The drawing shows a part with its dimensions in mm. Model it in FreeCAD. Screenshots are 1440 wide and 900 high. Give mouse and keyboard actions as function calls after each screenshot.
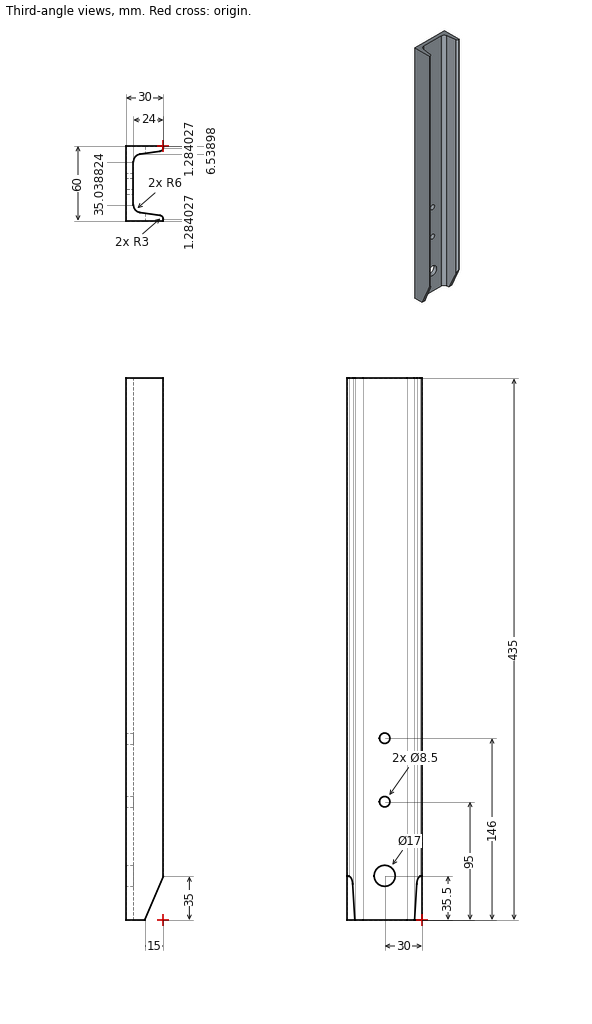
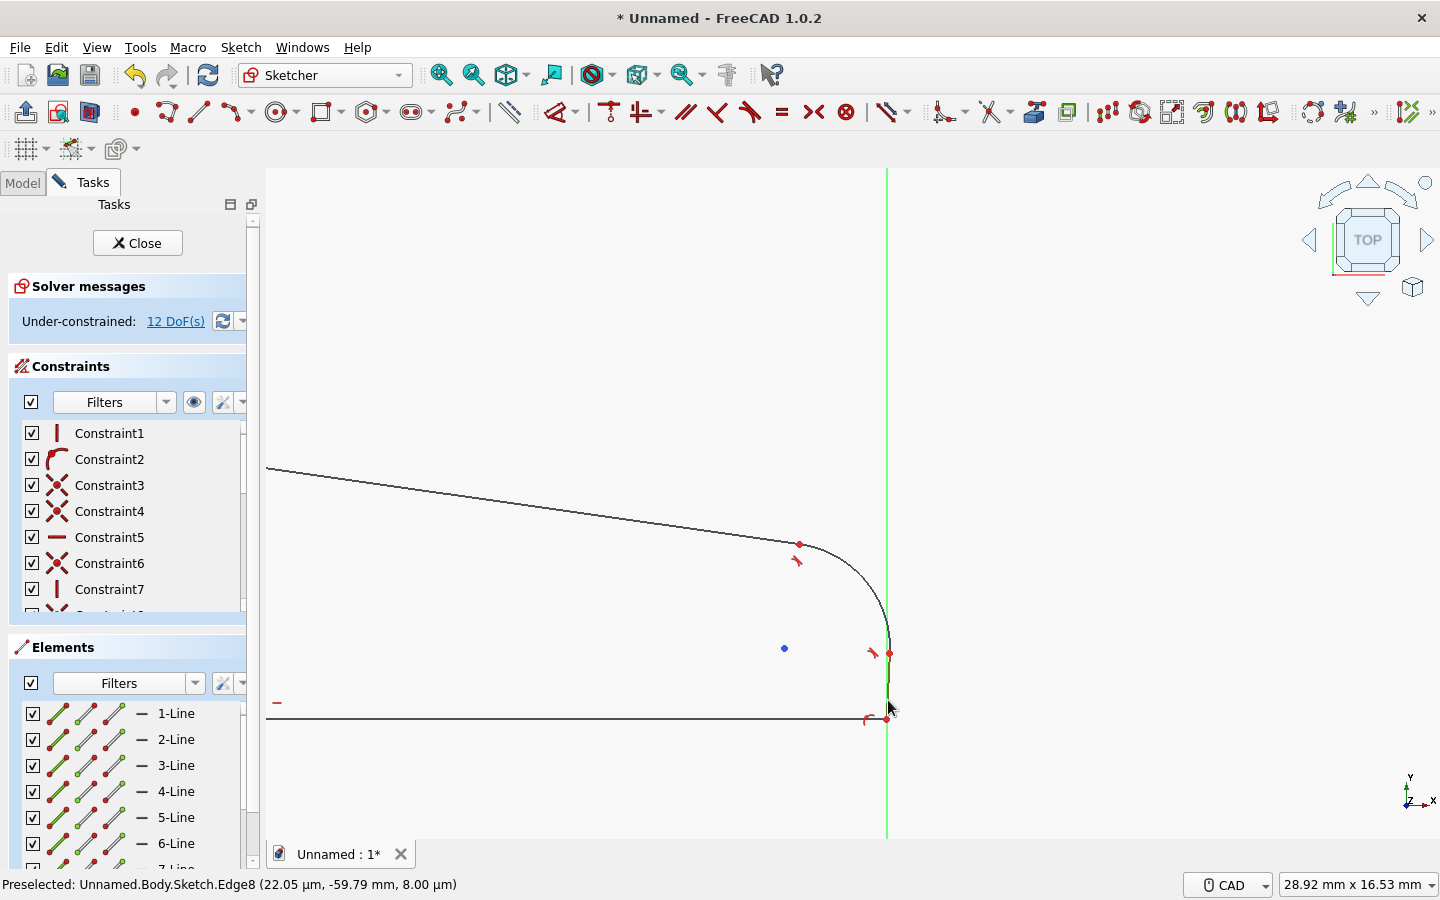
key(v)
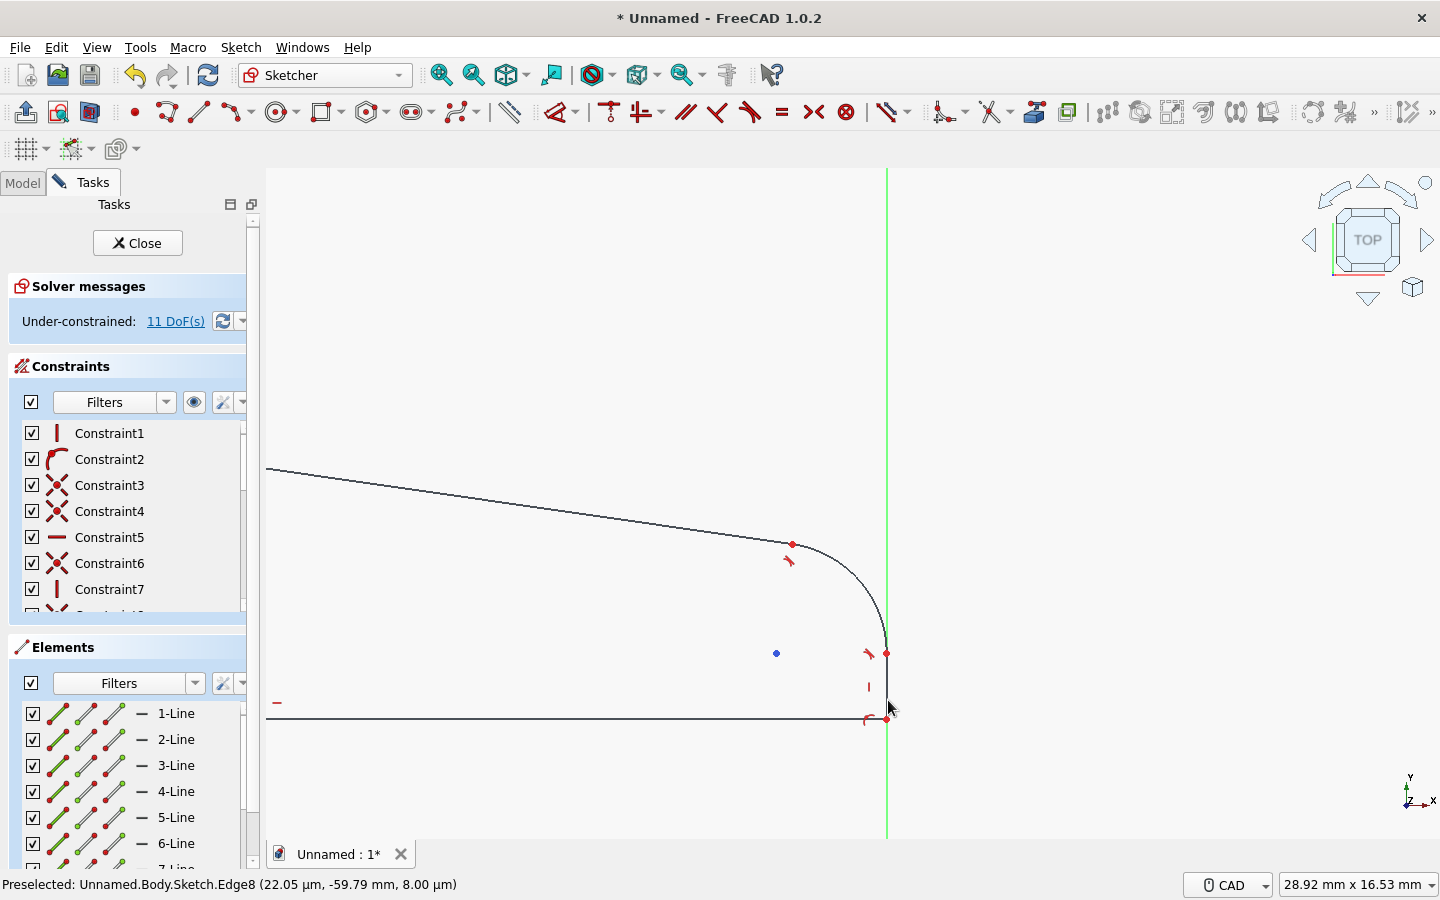
scroll(885, 704, down, 9)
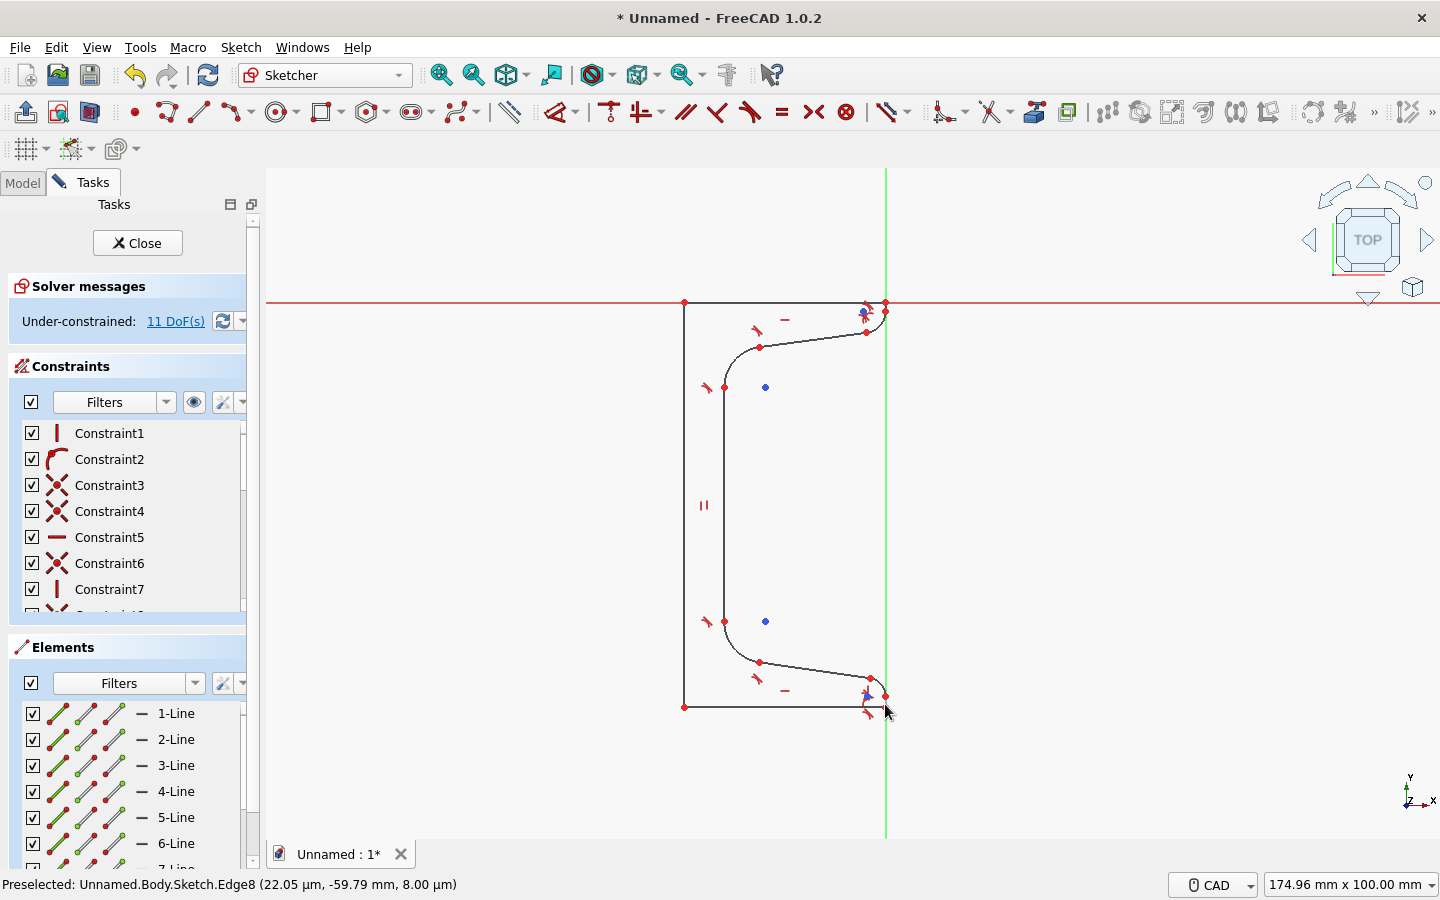
click(728, 639)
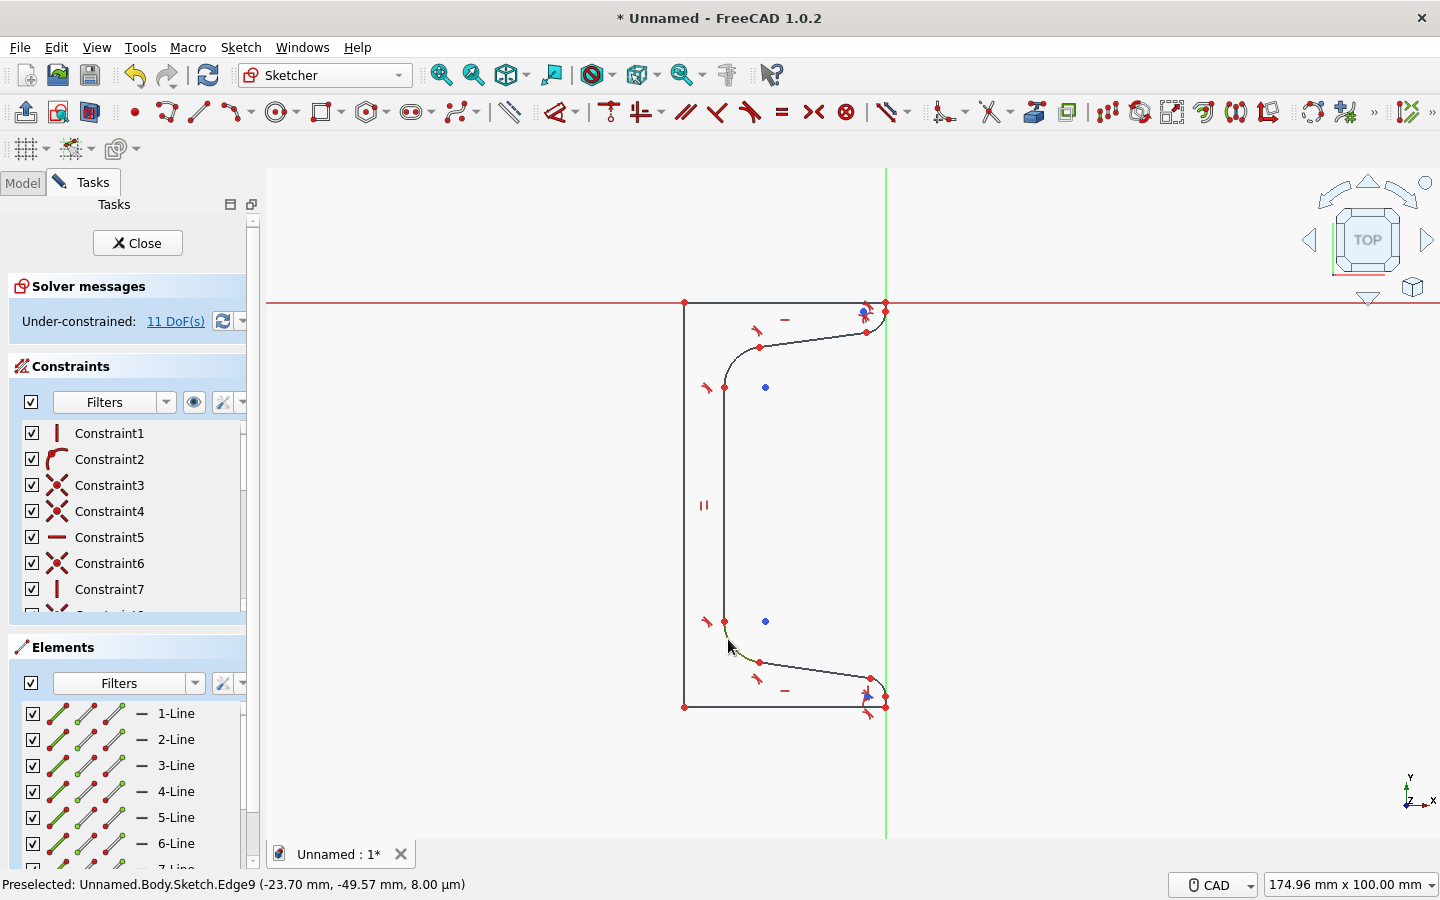
click(743, 353)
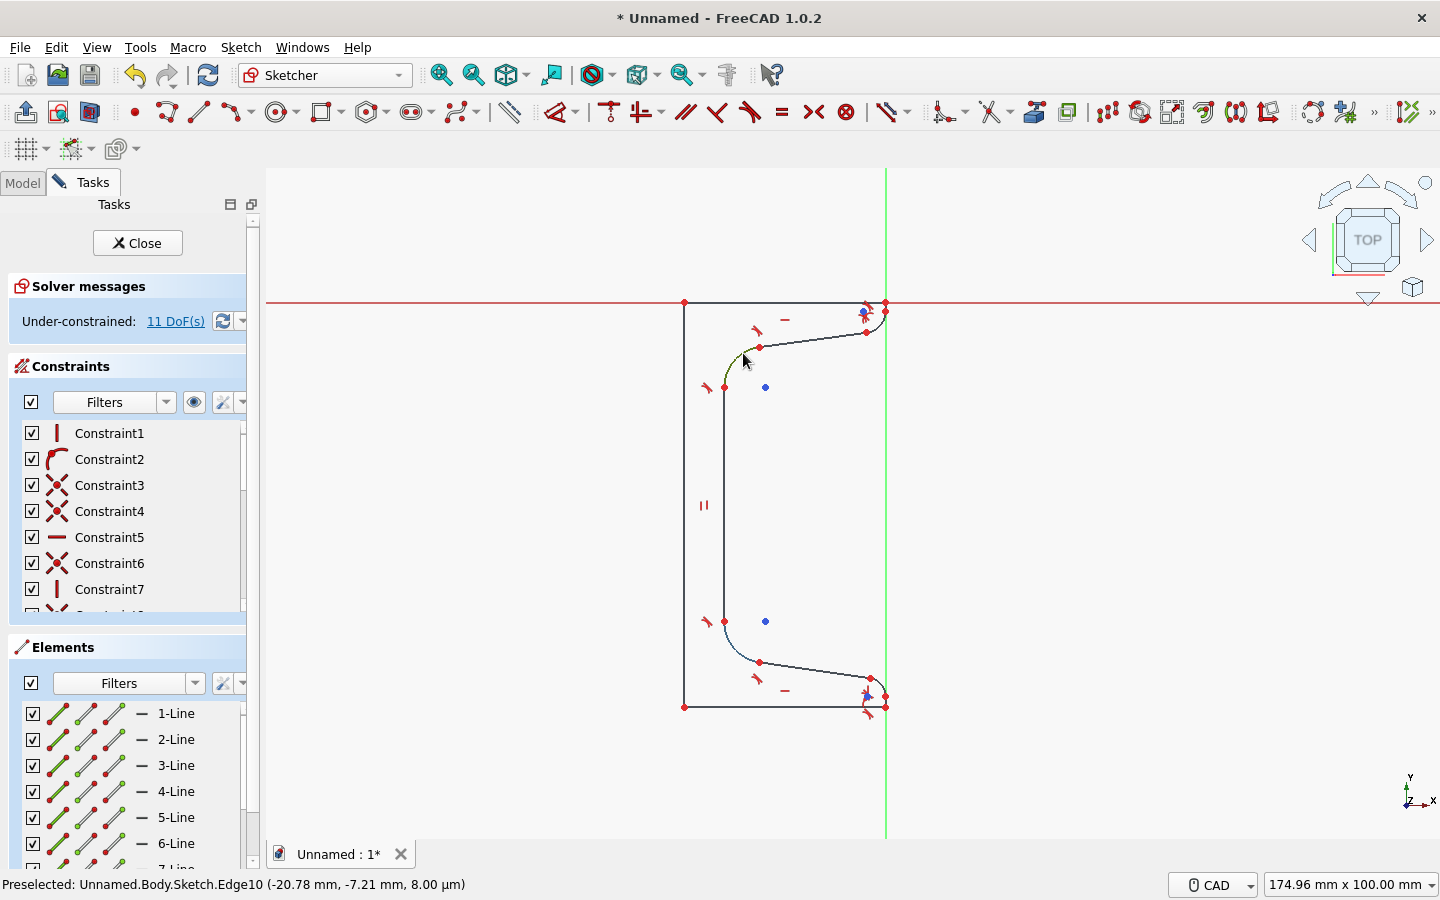
key(e)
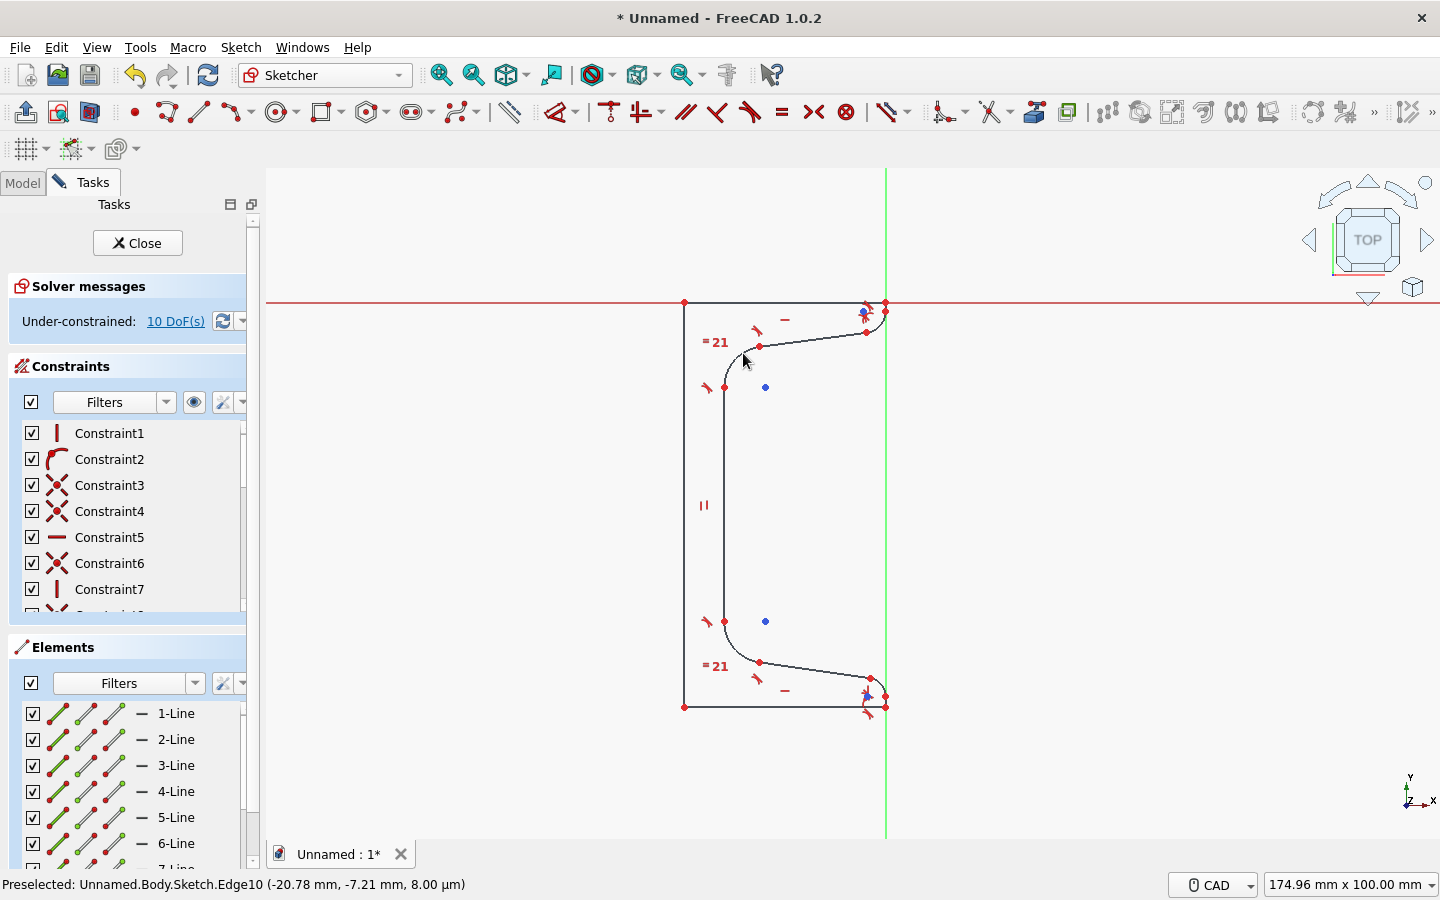
scroll(875, 330, up, 2)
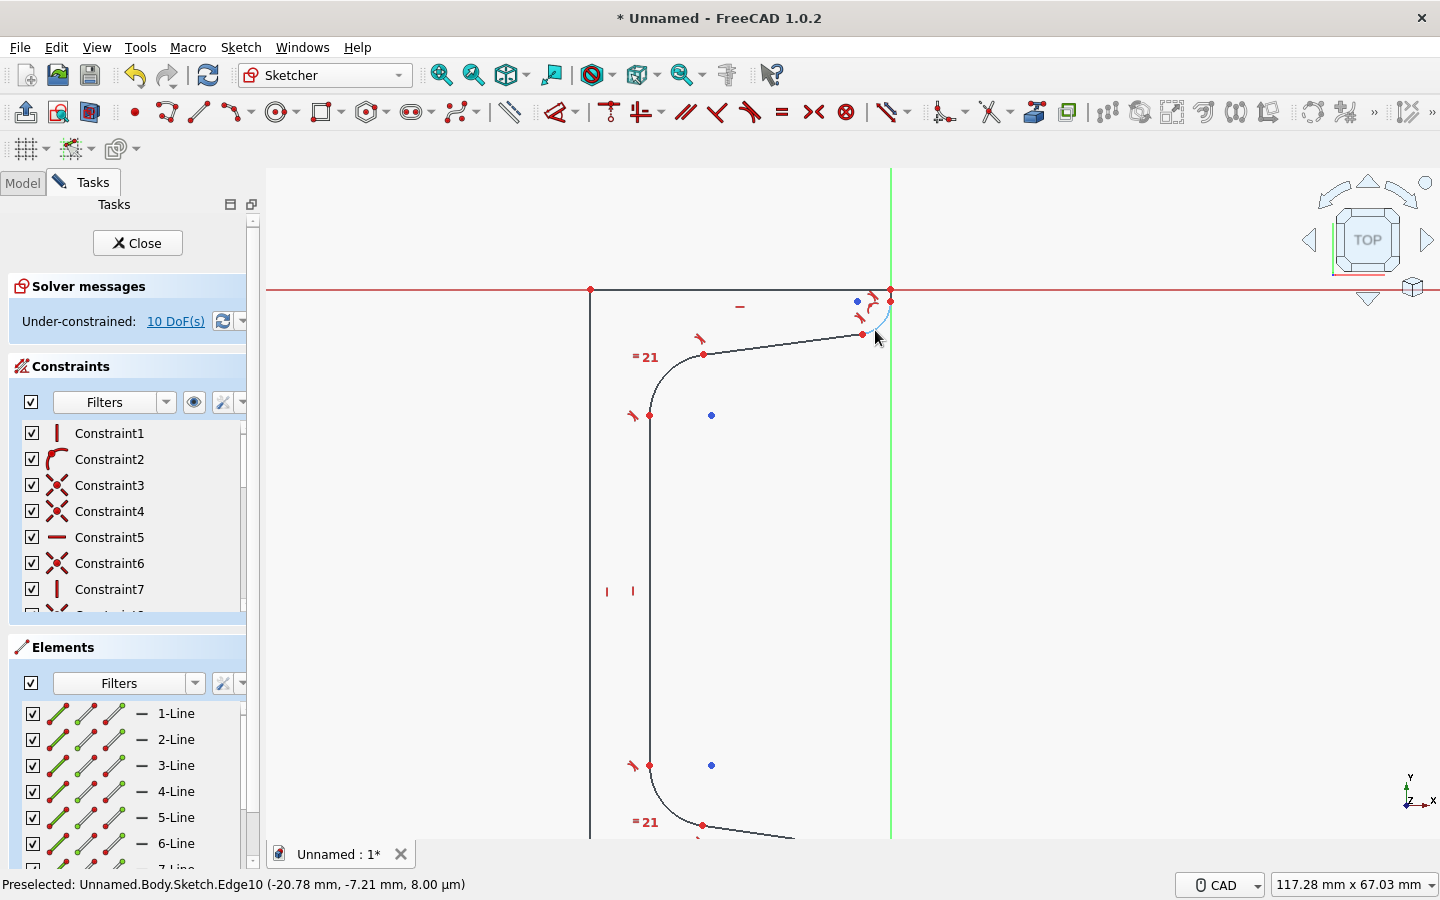
click(875, 329)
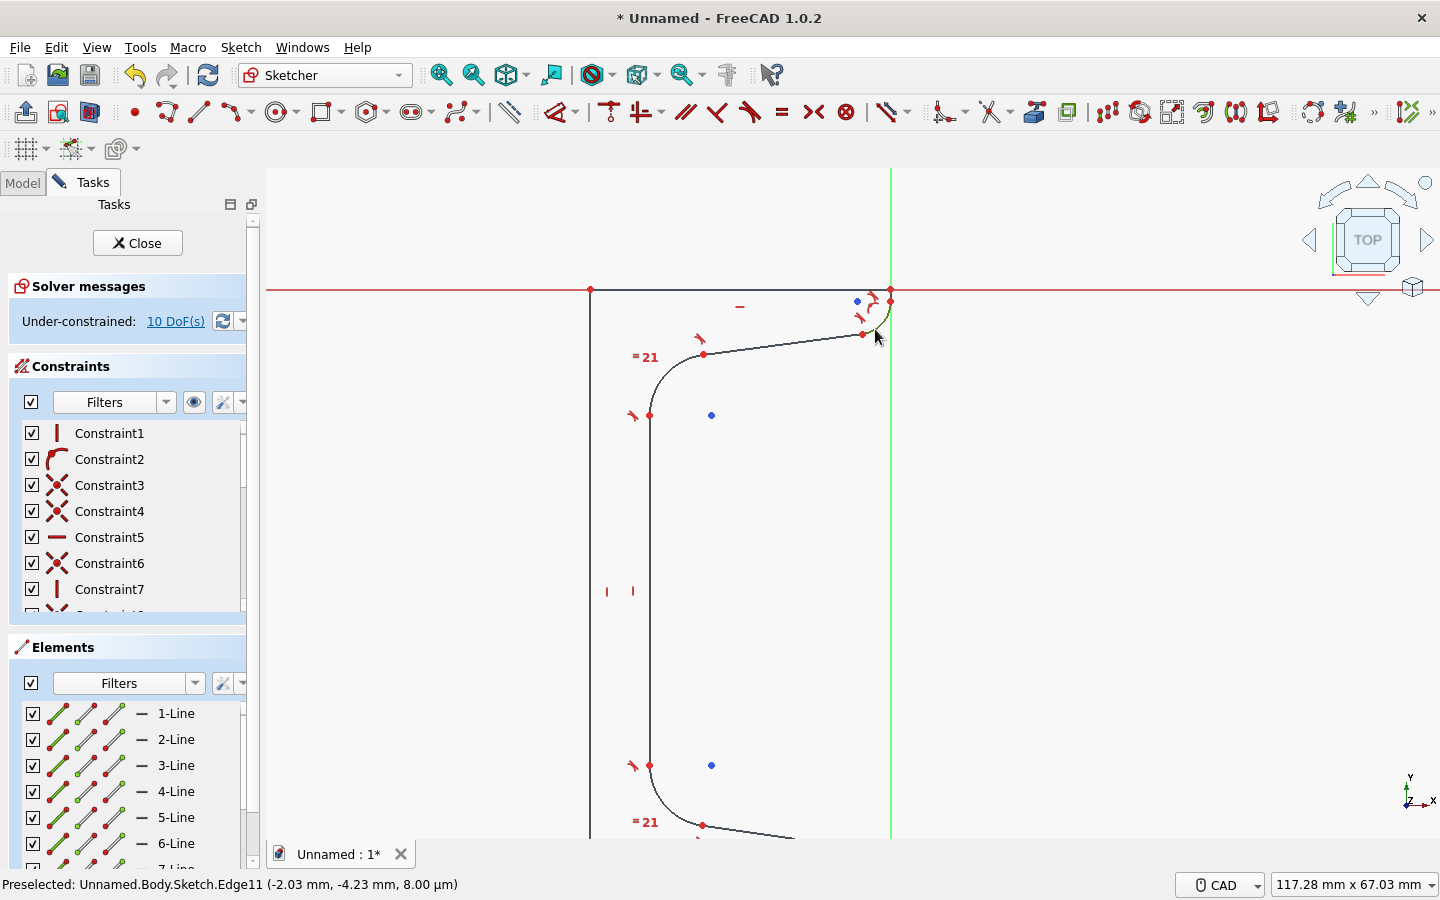
scroll(874, 328, down, 2)